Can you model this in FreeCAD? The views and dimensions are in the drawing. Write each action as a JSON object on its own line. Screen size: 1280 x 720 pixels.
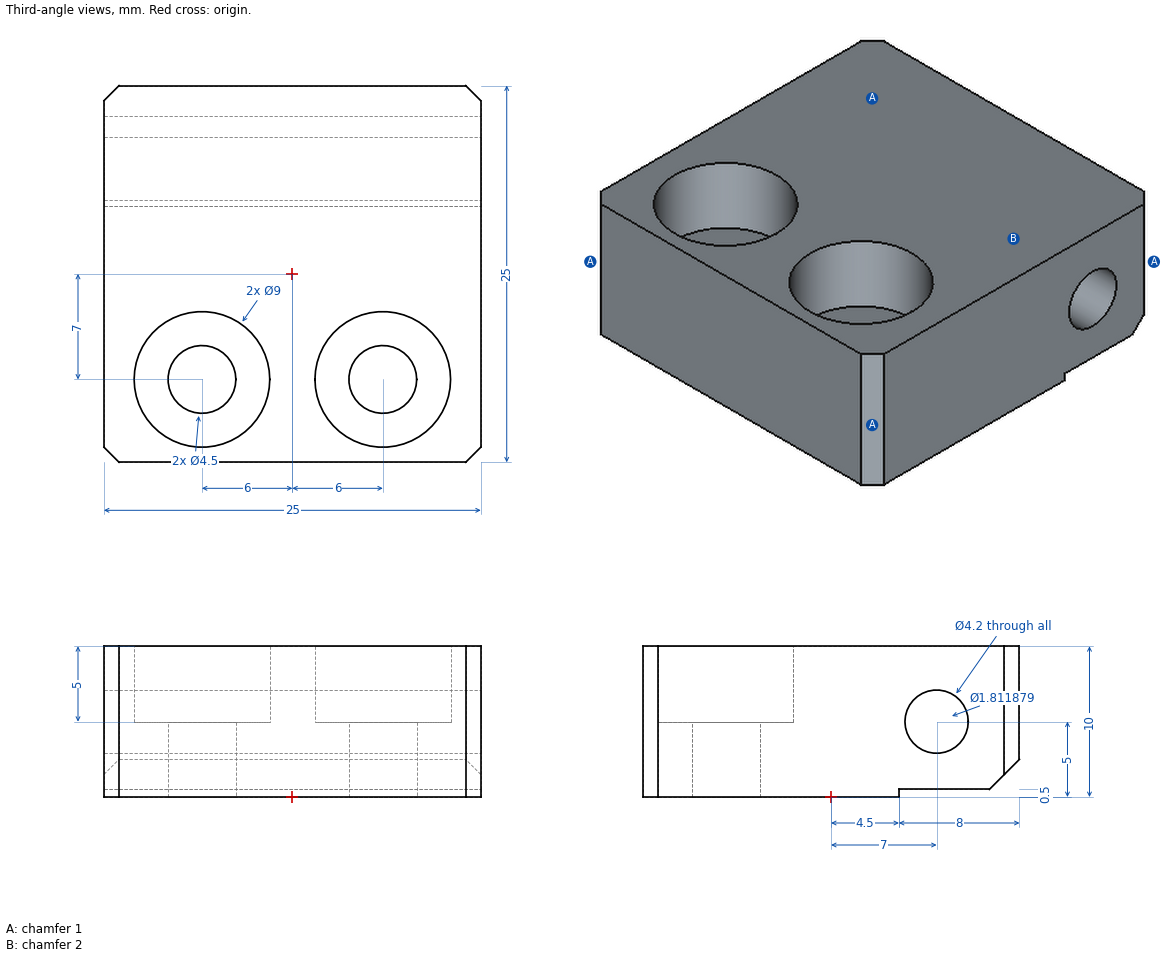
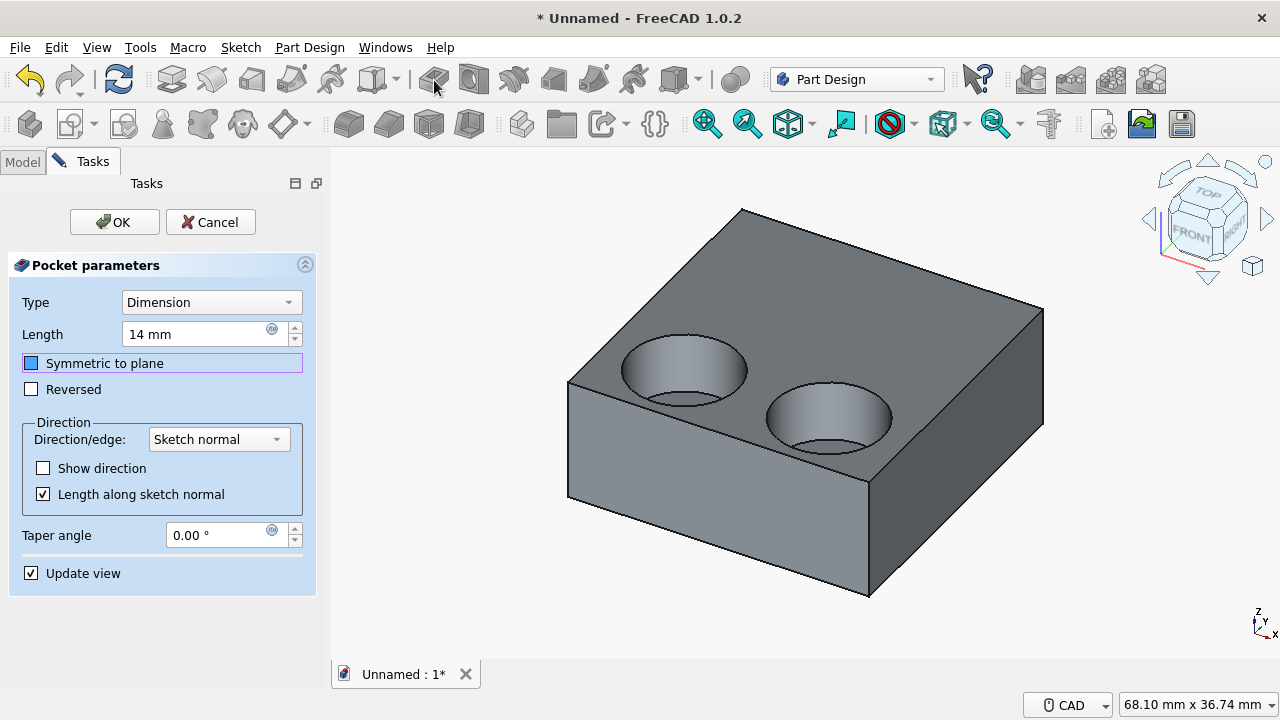
{"action": "left_click", "coordinate": [115, 222]}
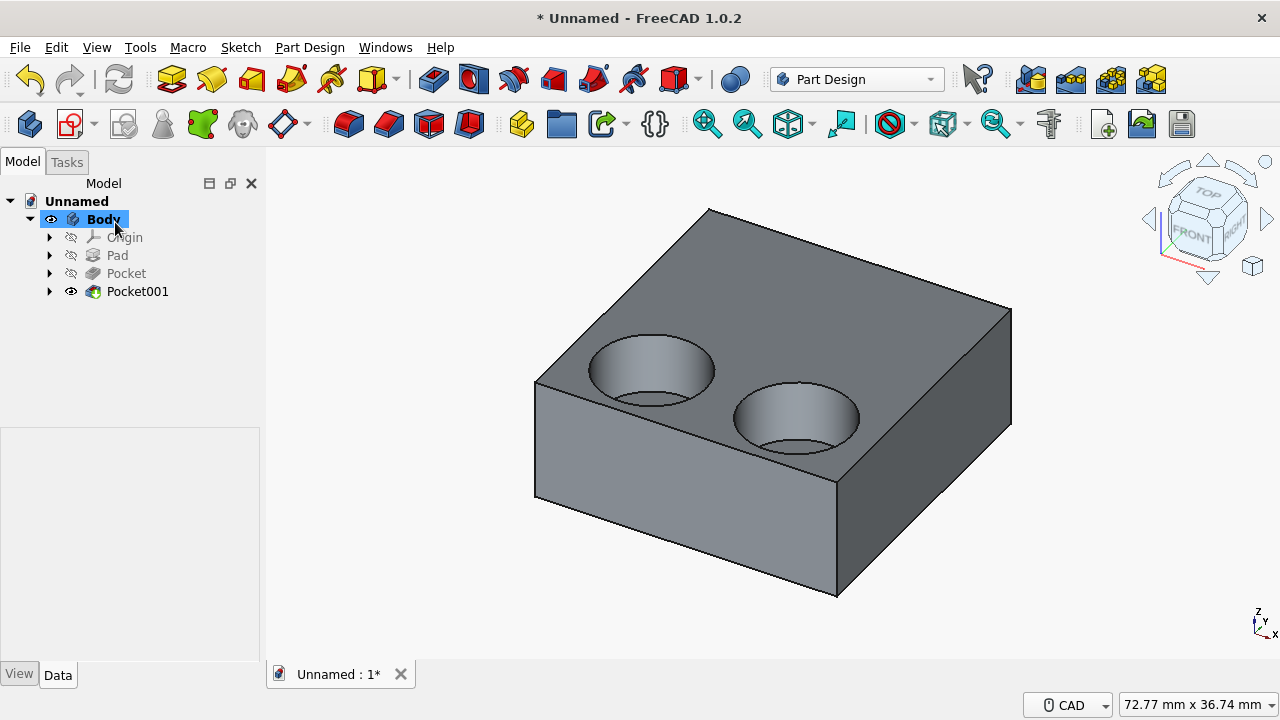
{"action": "key", "text": "6"}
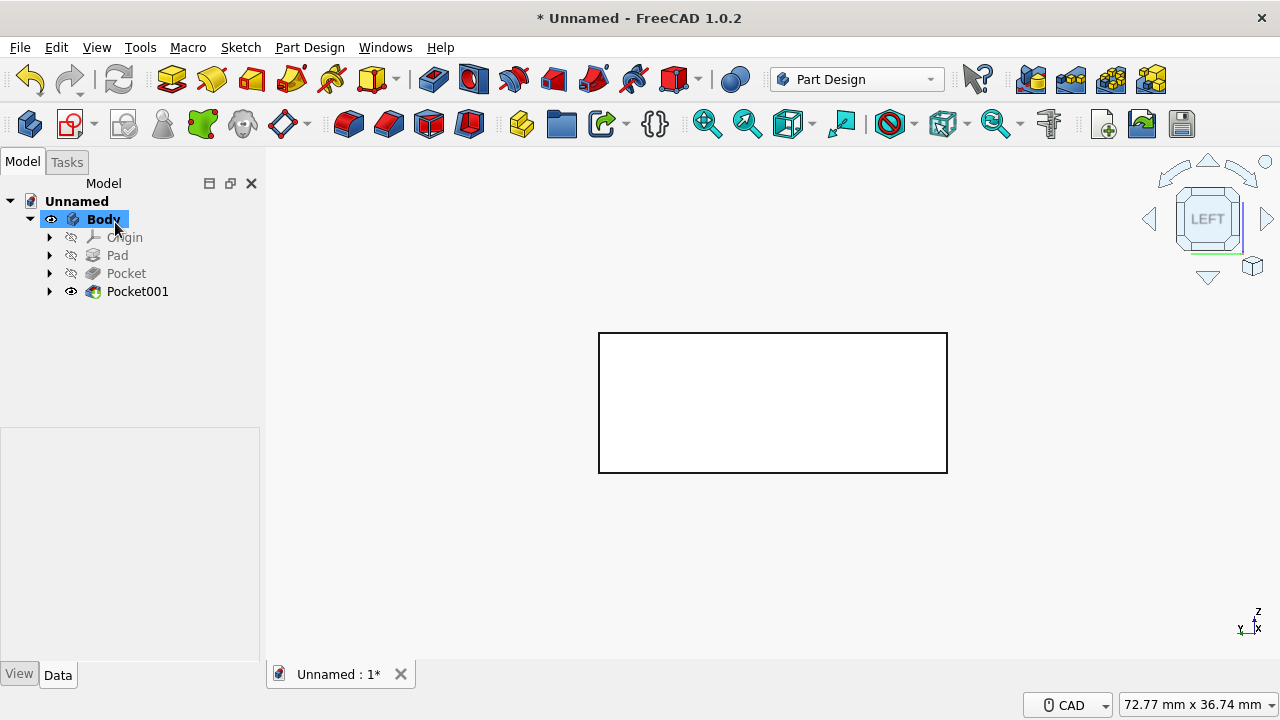
{"action": "key", "text": "v f"}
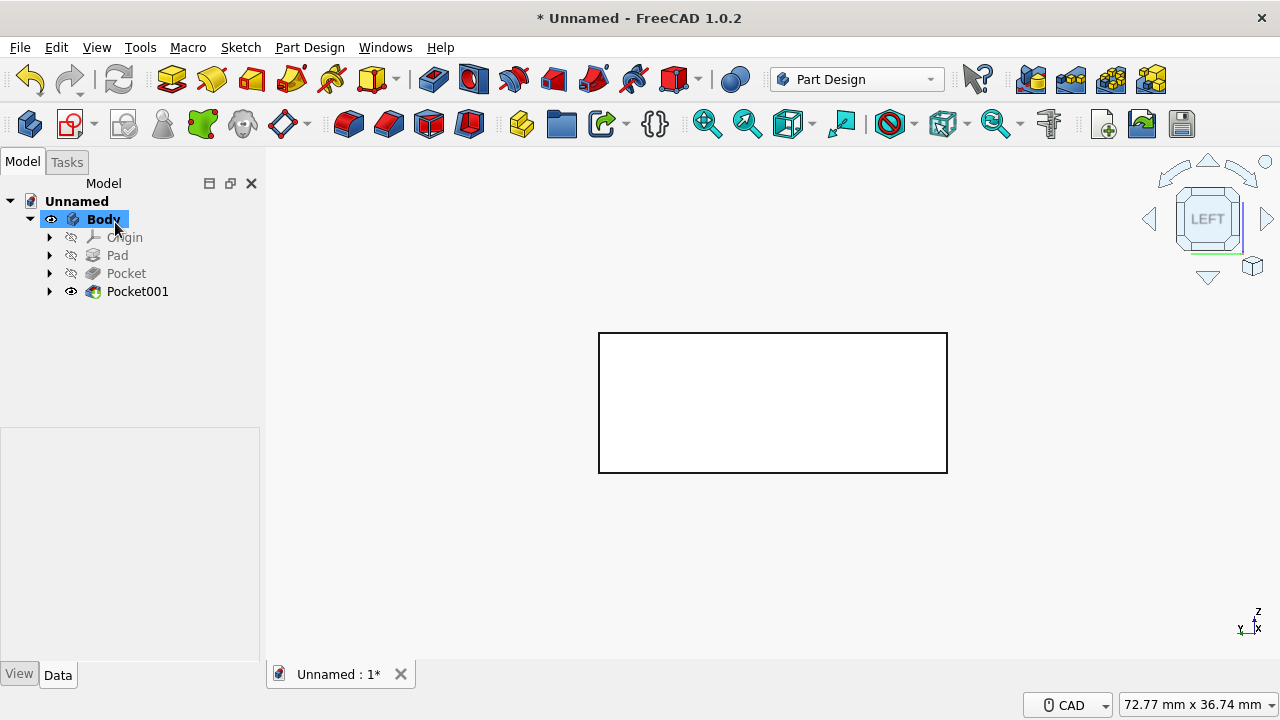
{"action": "left_click", "coordinate": [673, 402]}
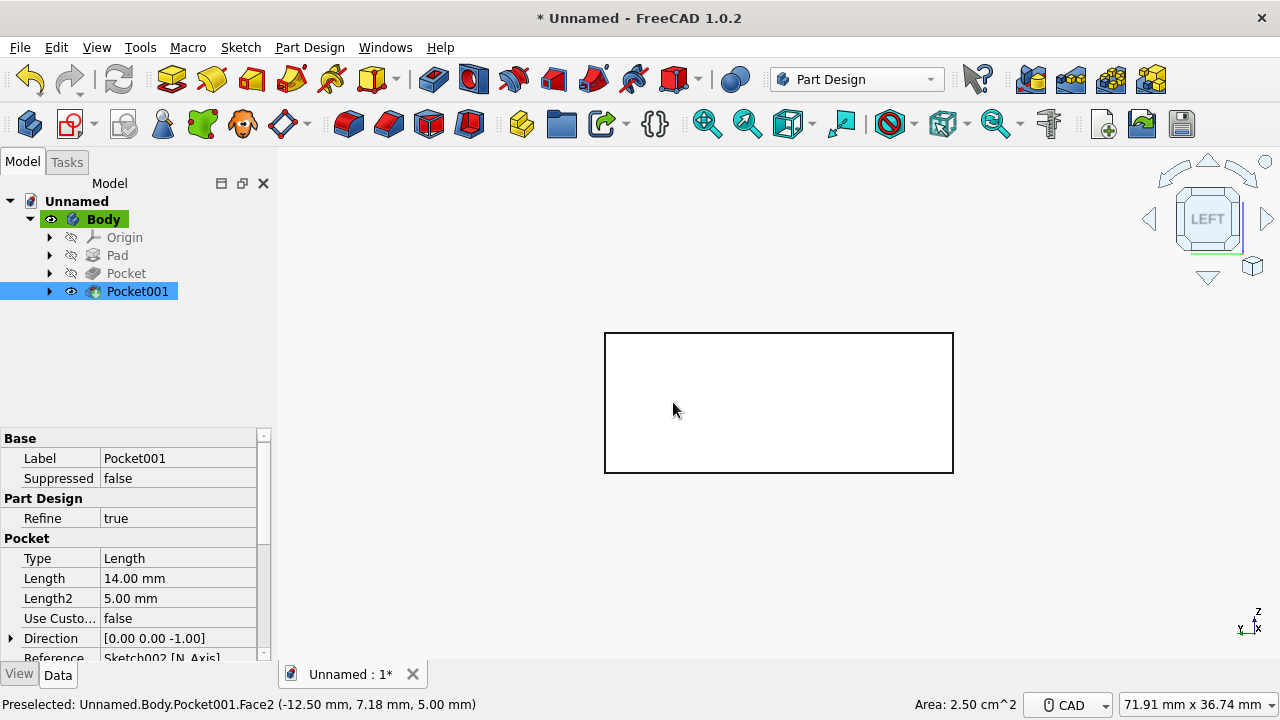
{"action": "left_click", "coordinate": [70, 124]}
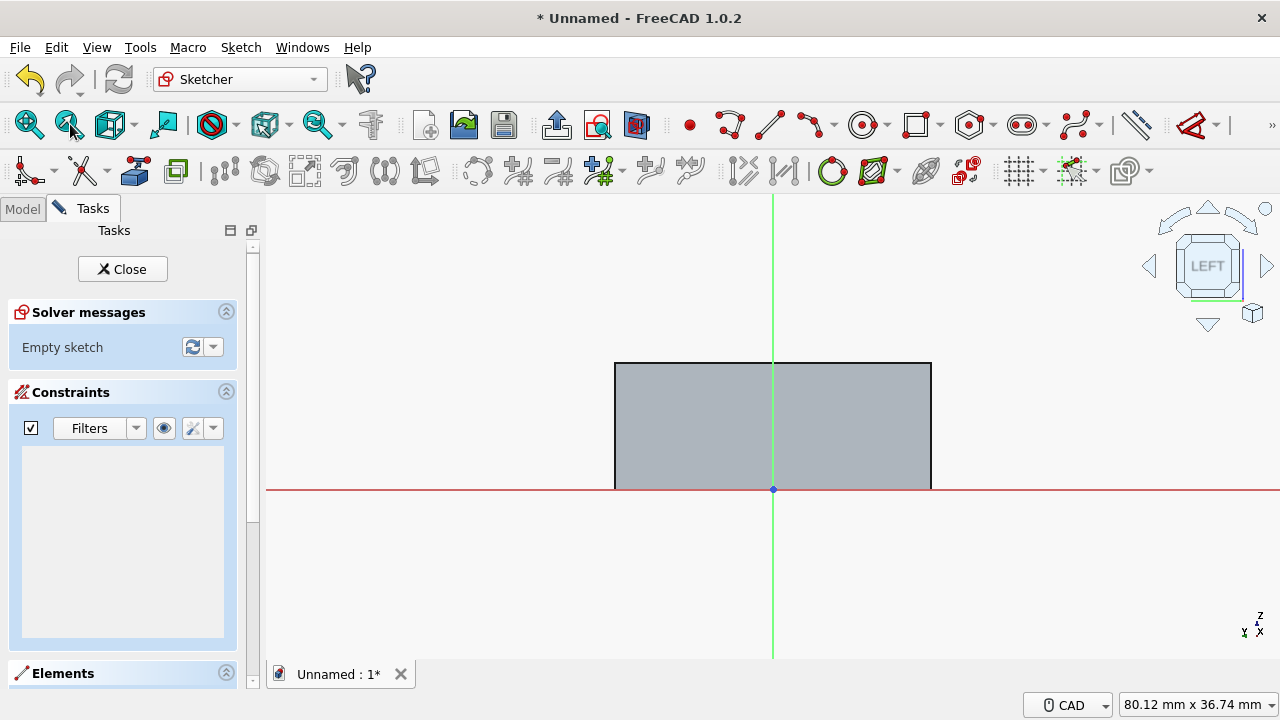
{"action": "scroll", "coordinate": [683, 426], "scroll_direction": "up", "scroll_amount": 13}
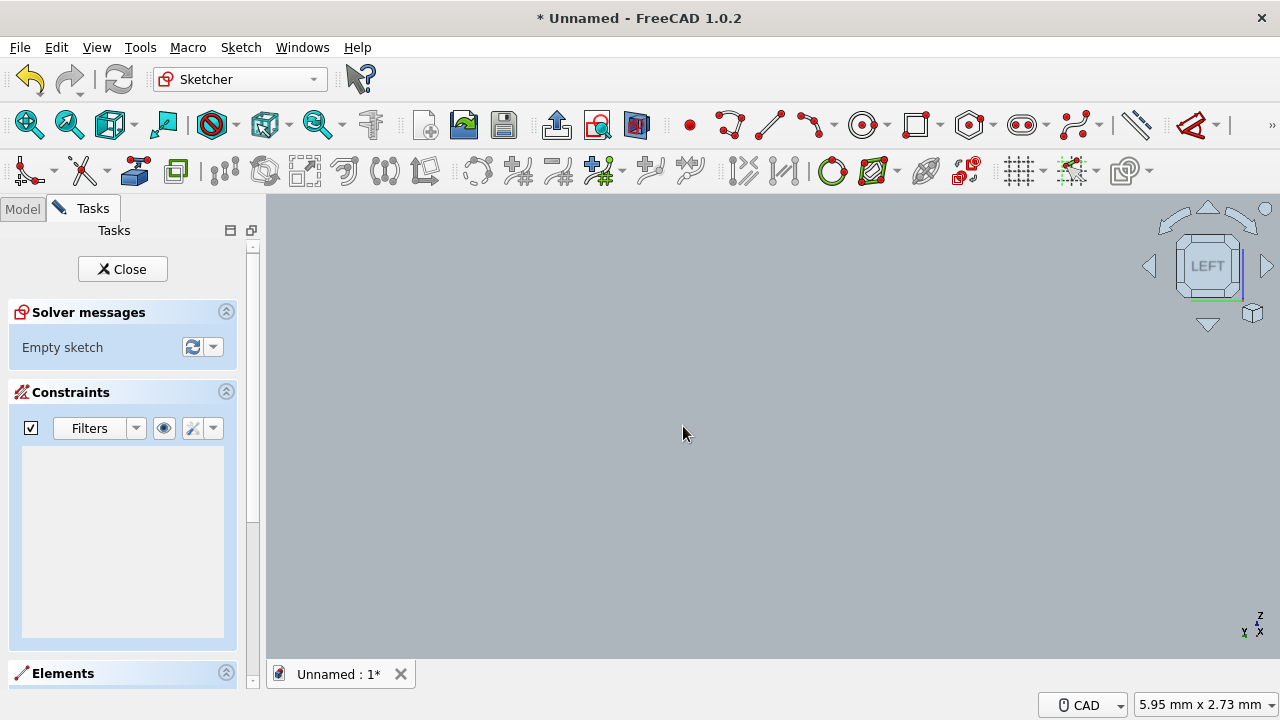
{"action": "key", "text": "g c"}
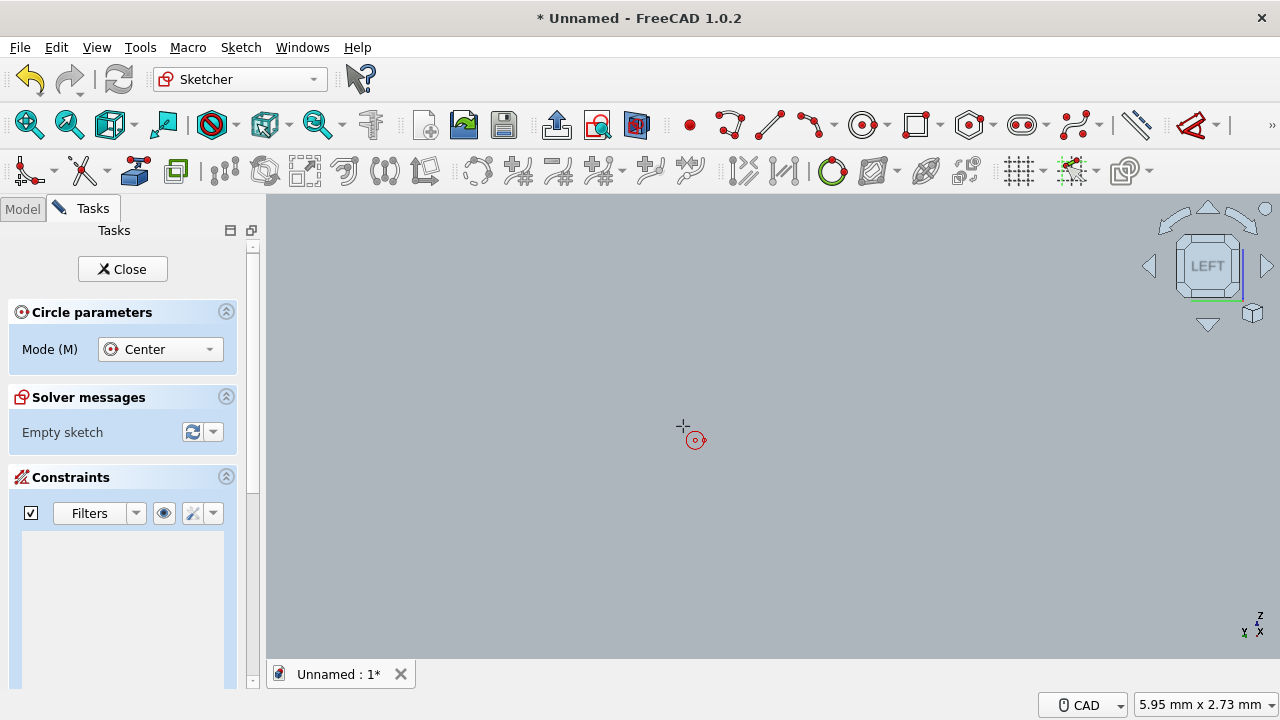
{"action": "left_click", "coordinate": [697, 427]}
{"action": "left_click", "coordinate": [806, 317]}
{"action": "key", "text": "Escape"}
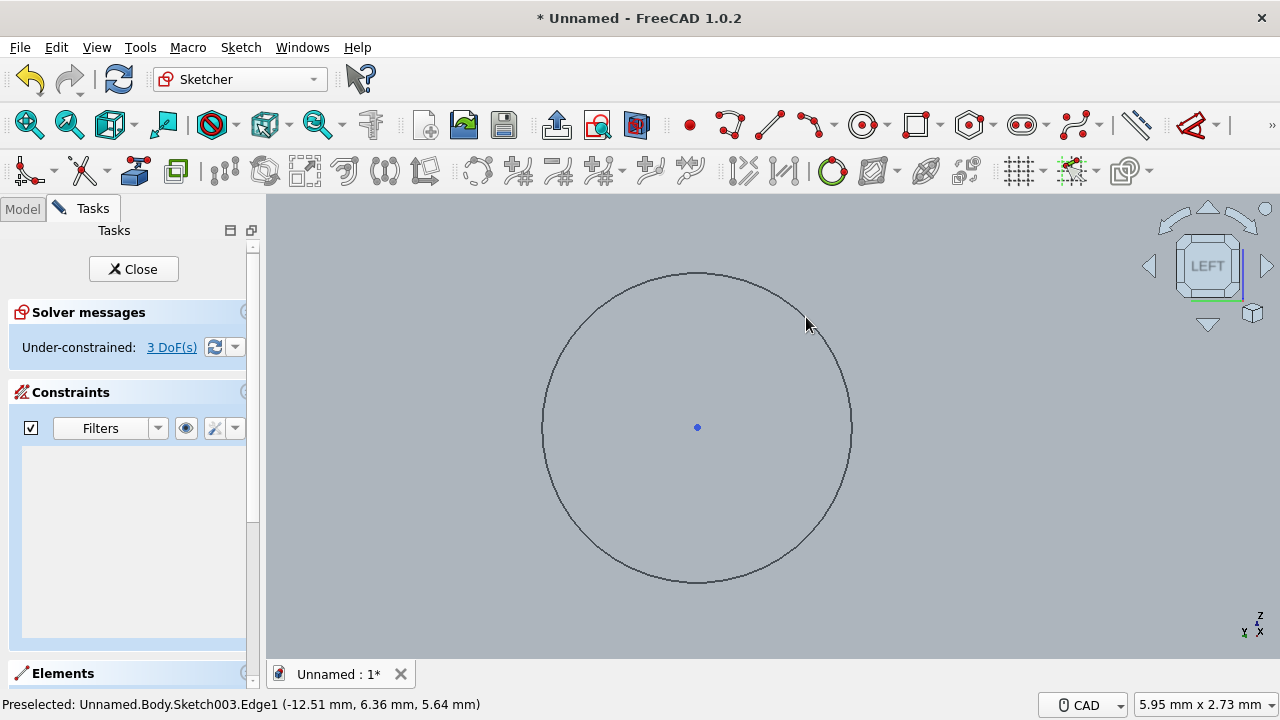
{"action": "key", "text": "d"}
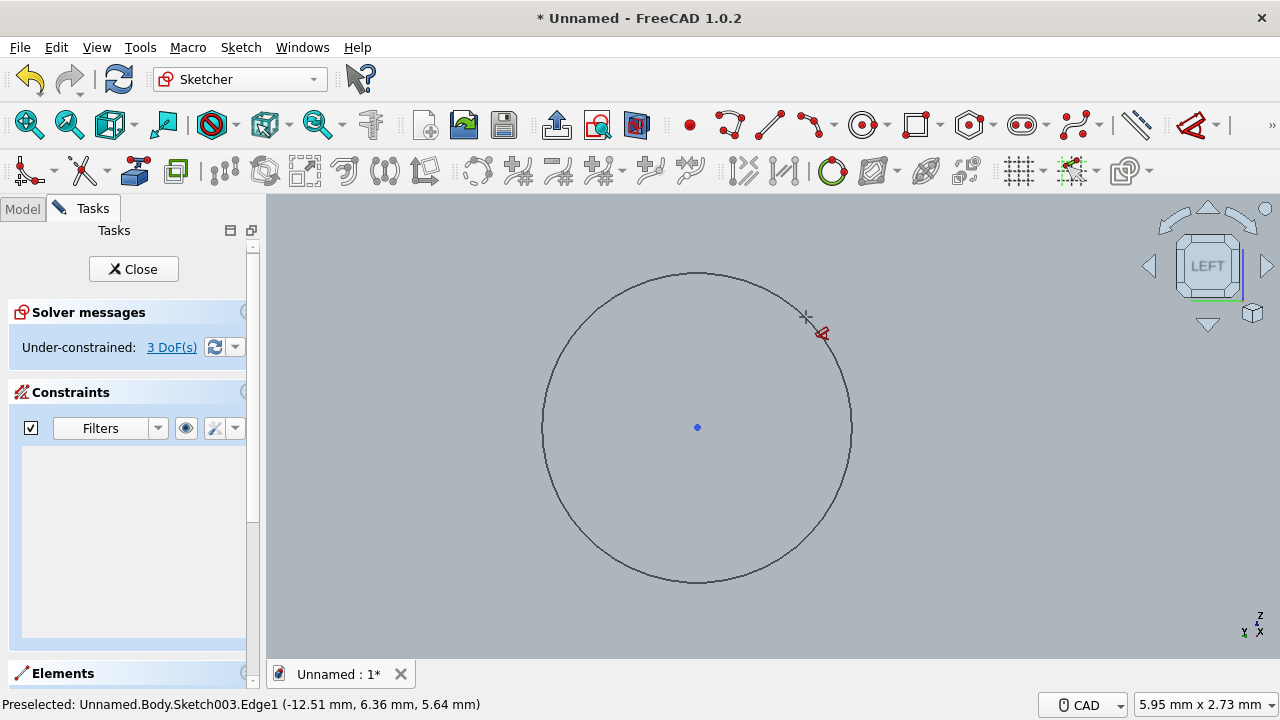
{"action": "left_click", "coordinate": [806, 318]}
{"action": "left_click", "coordinate": [829, 295]}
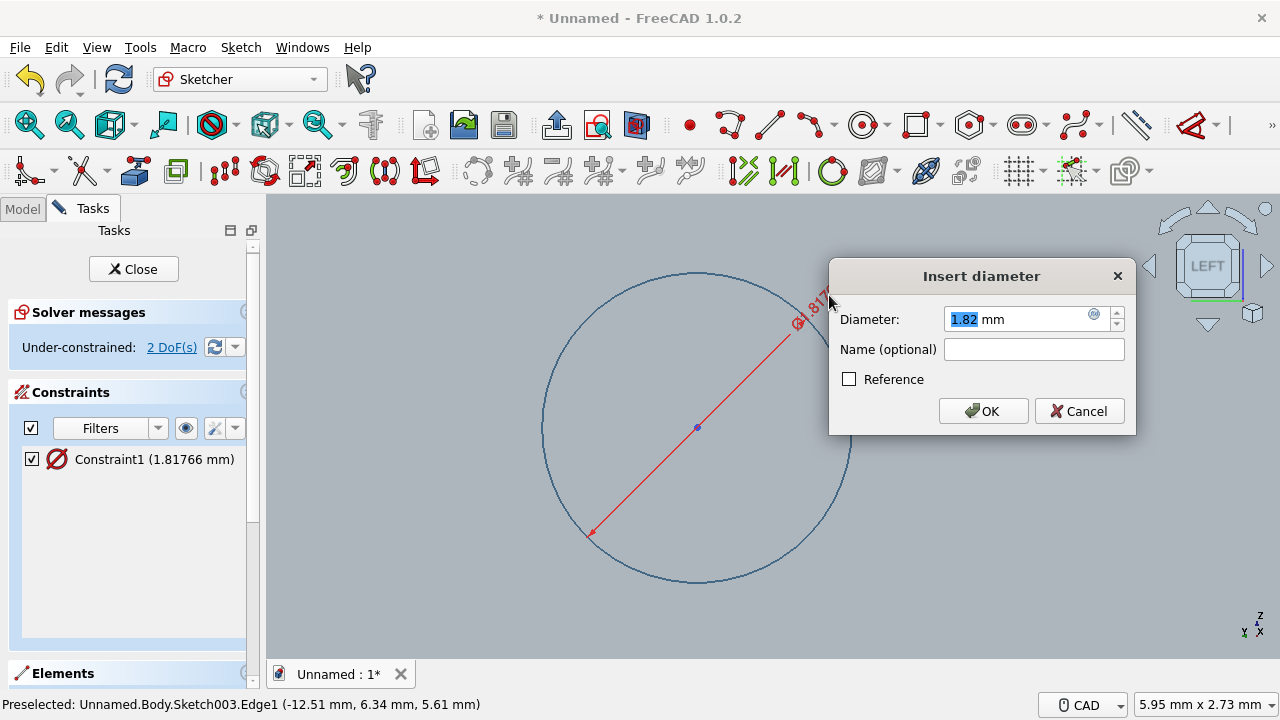
{"action": "type", "text": "1.811879"}
{"action": "key", "text": "Return"}